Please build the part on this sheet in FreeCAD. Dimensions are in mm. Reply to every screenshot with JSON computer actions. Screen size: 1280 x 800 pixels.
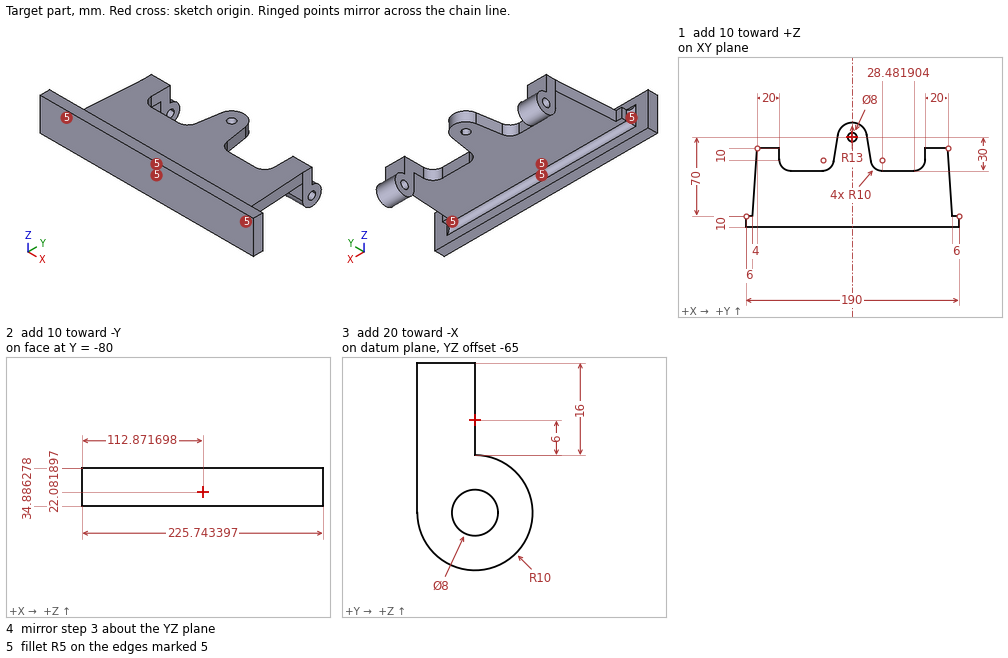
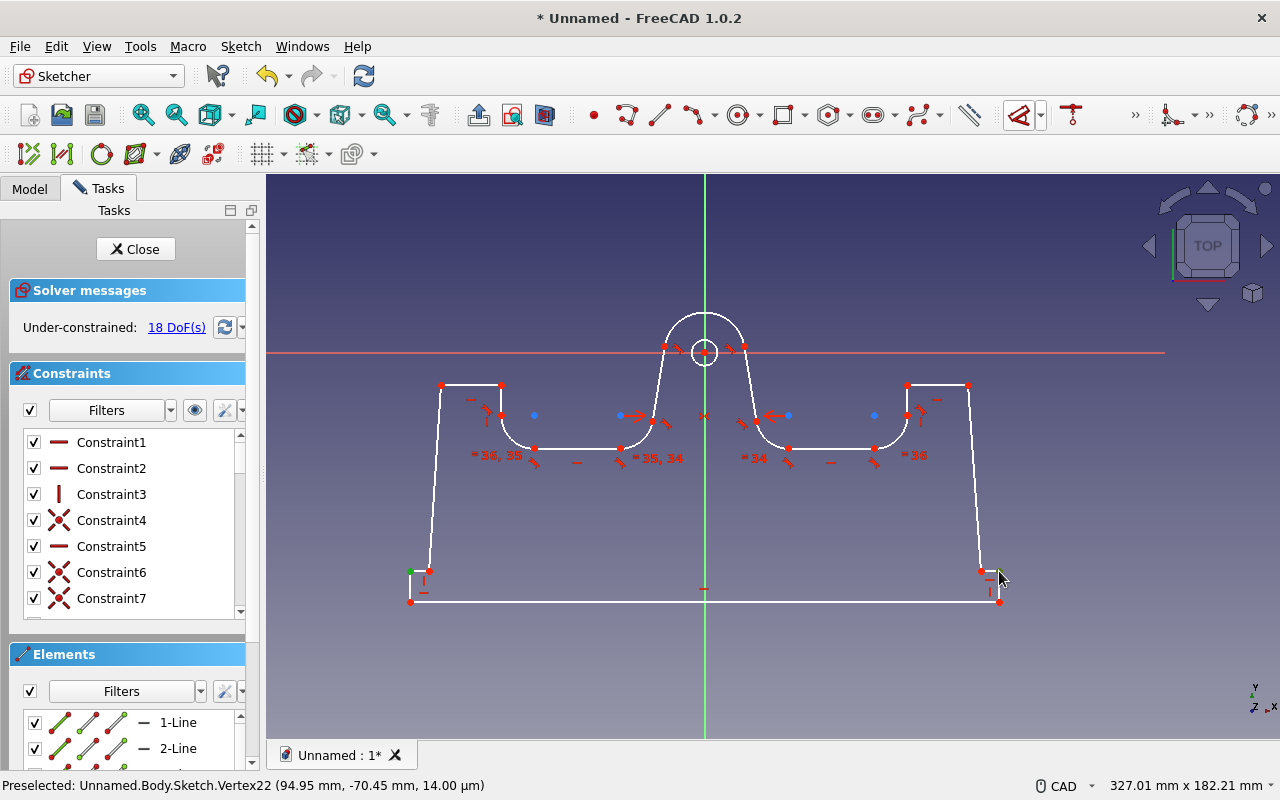
{"action": "left_click", "coordinate": [705, 675]}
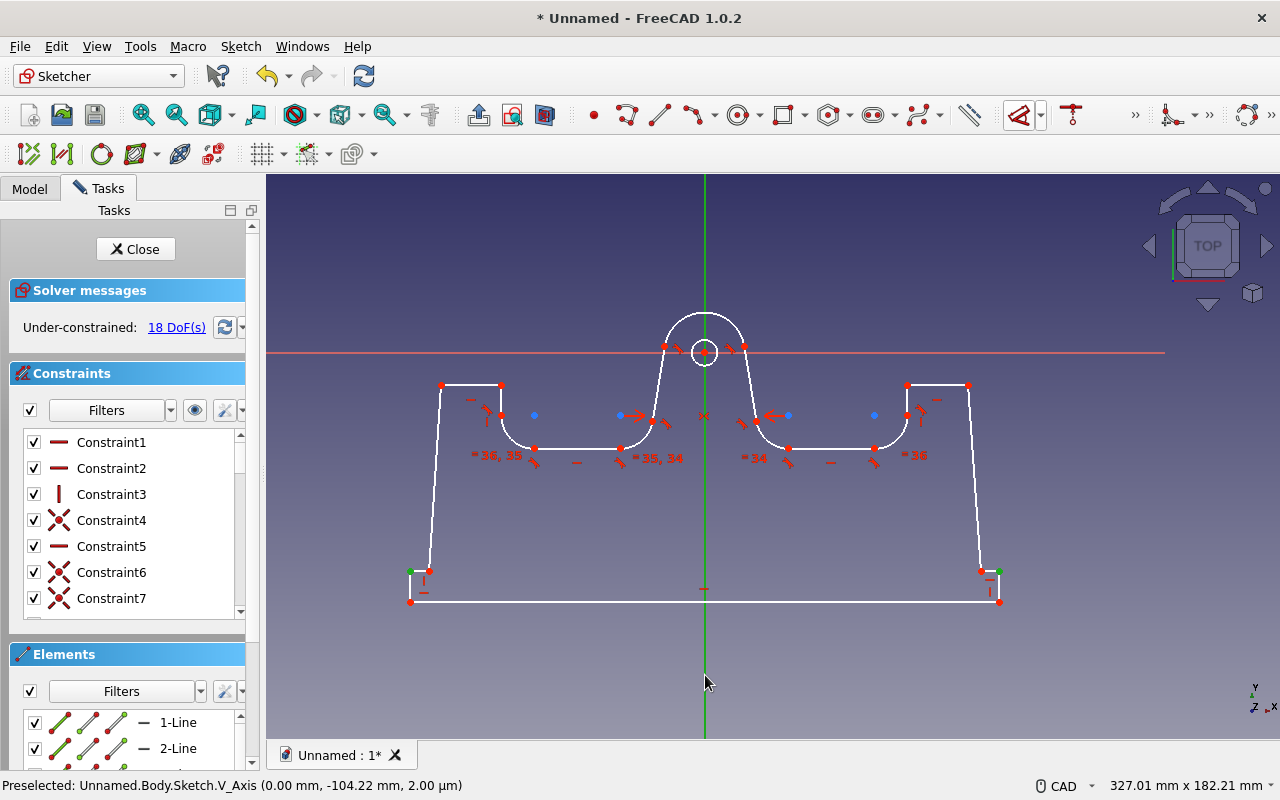
{"action": "key", "text": "s"}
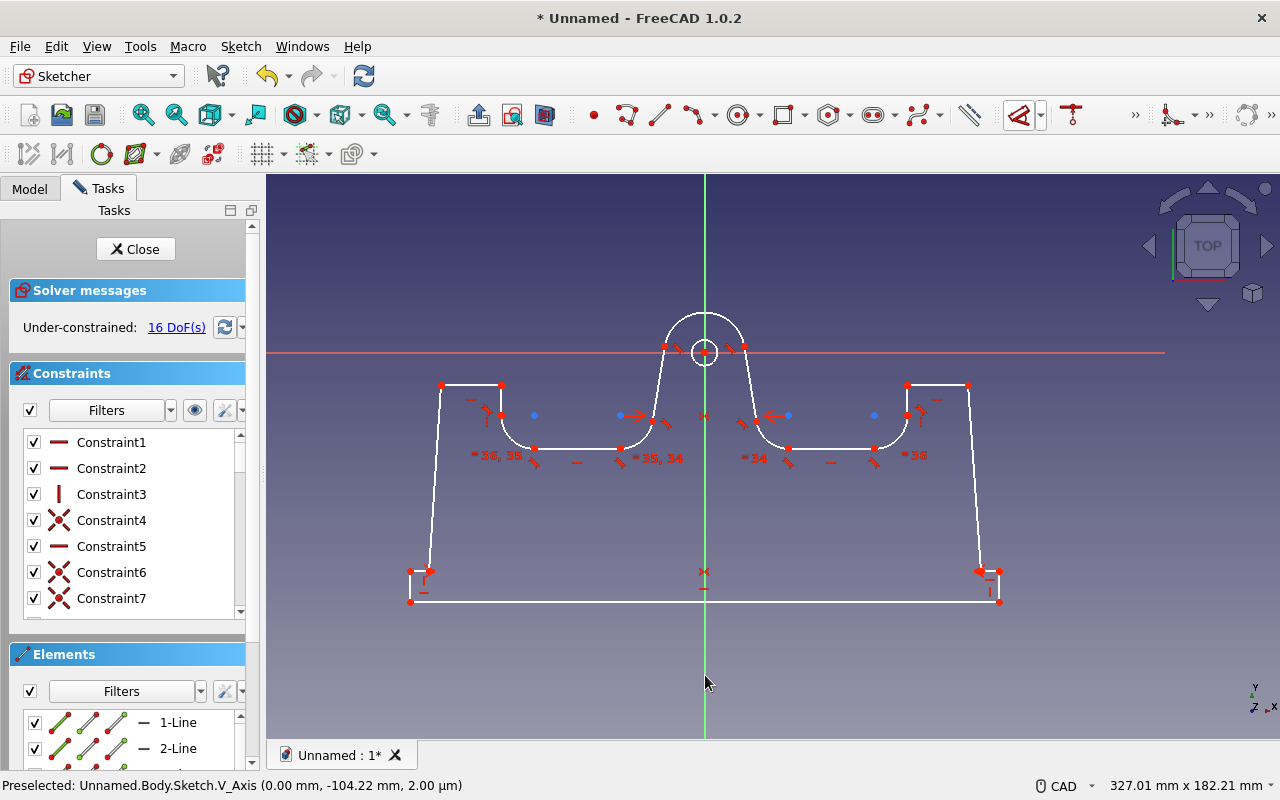
{"action": "left_click", "coordinate": [441, 385]}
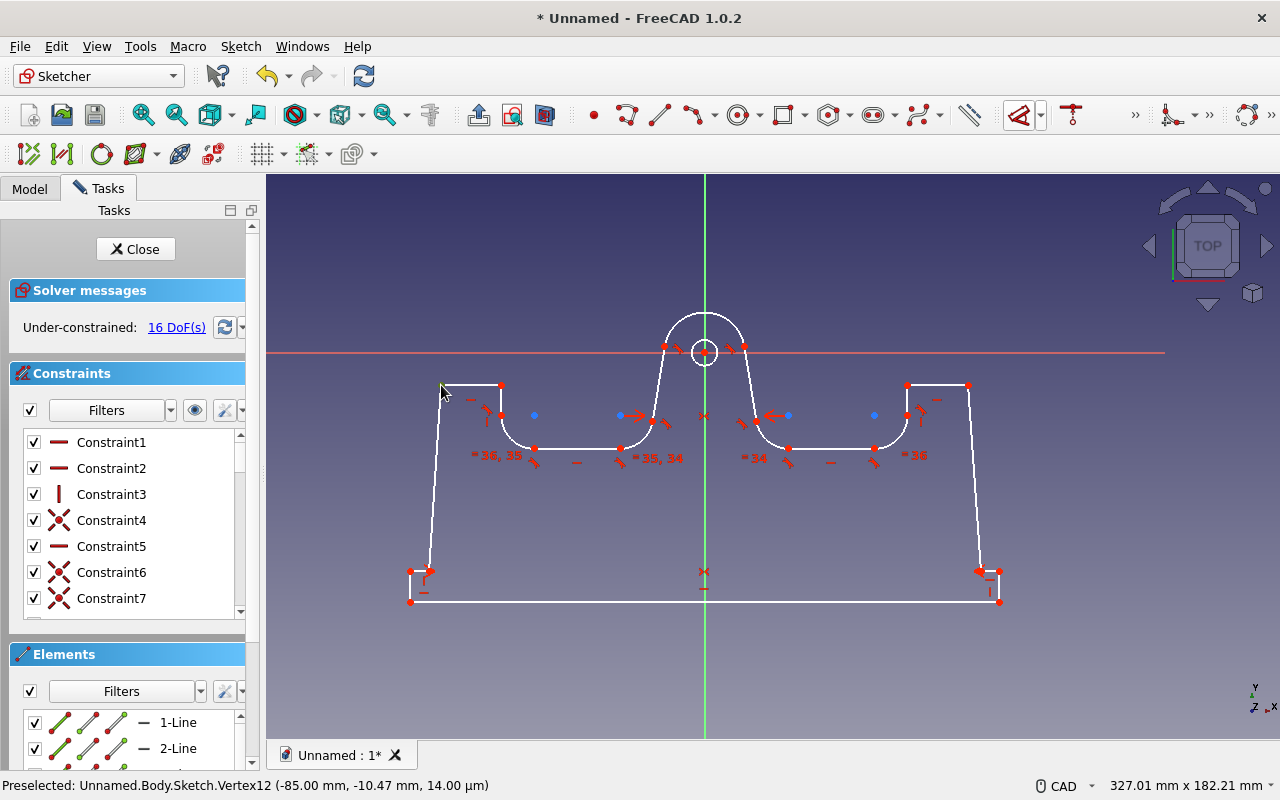
{"action": "left_click", "coordinate": [968, 385]}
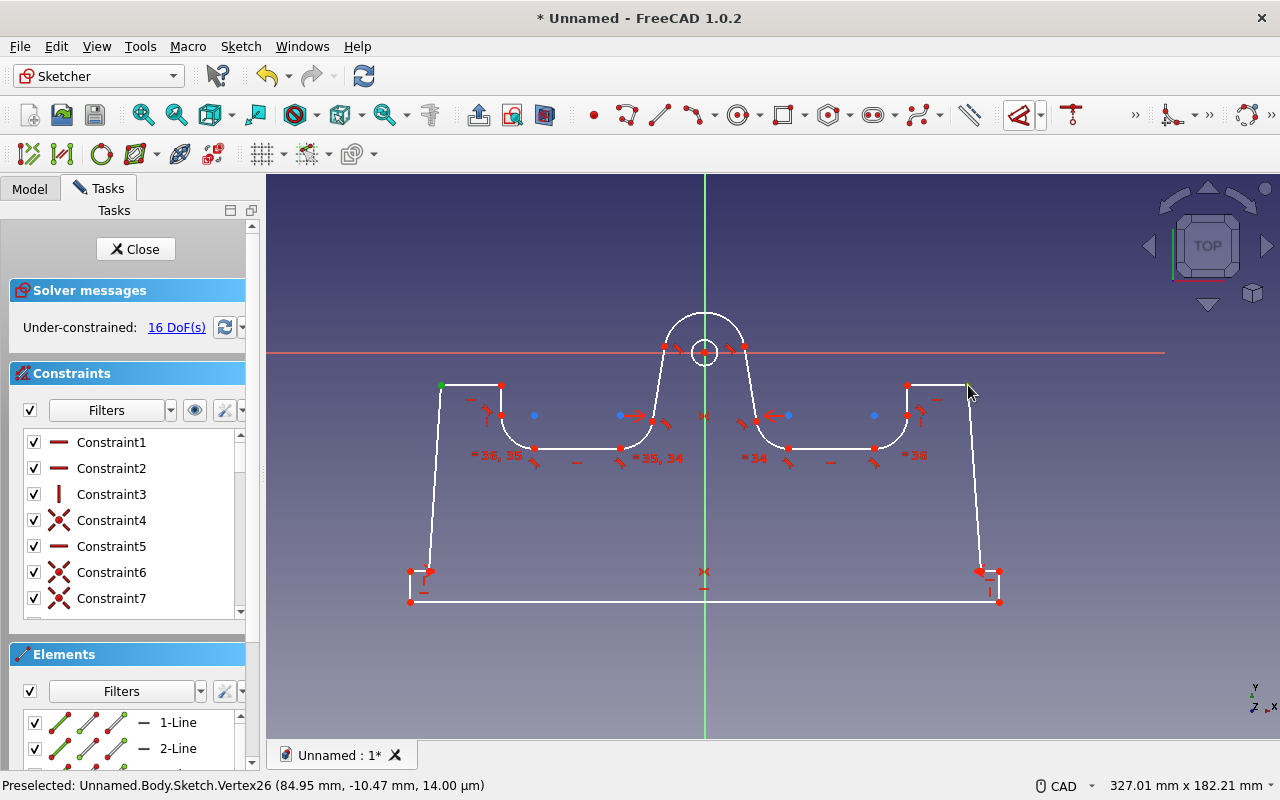
{"action": "left_click", "coordinate": [705, 675]}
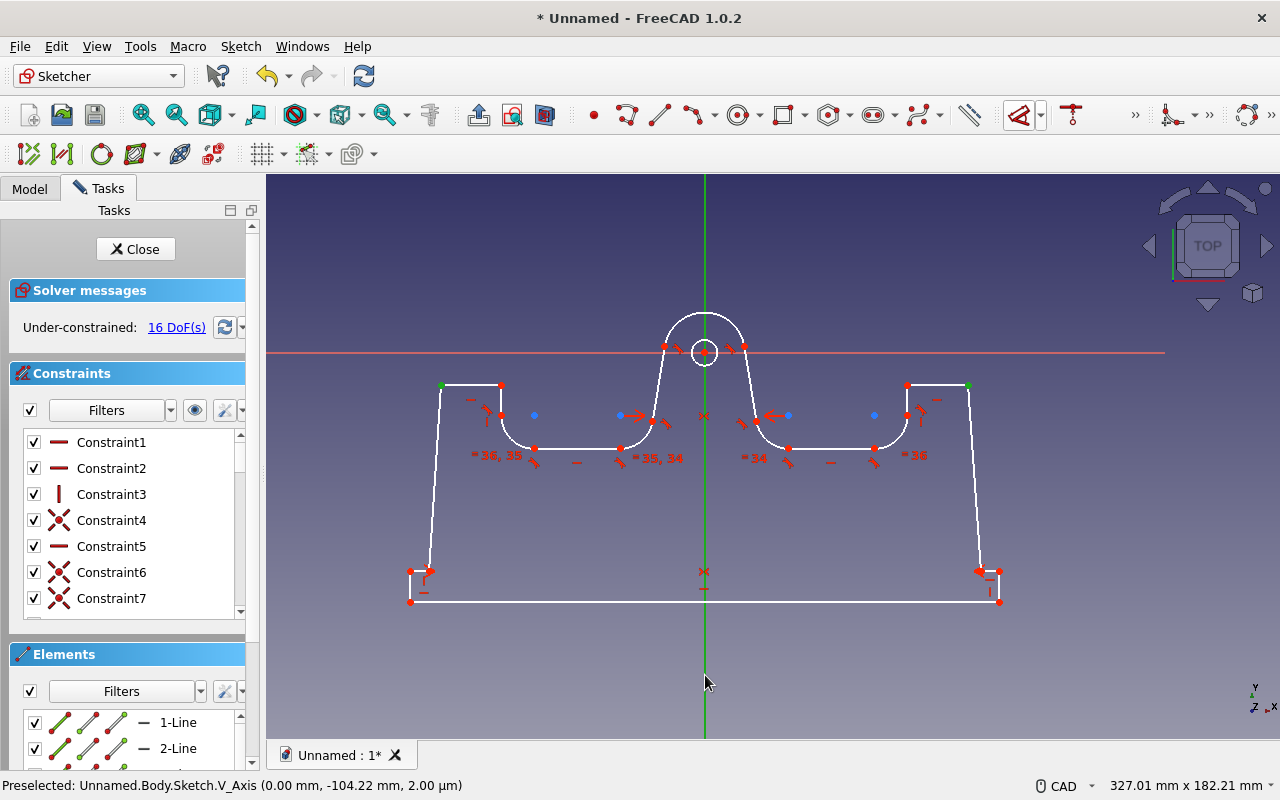
{"action": "key", "text": "s"}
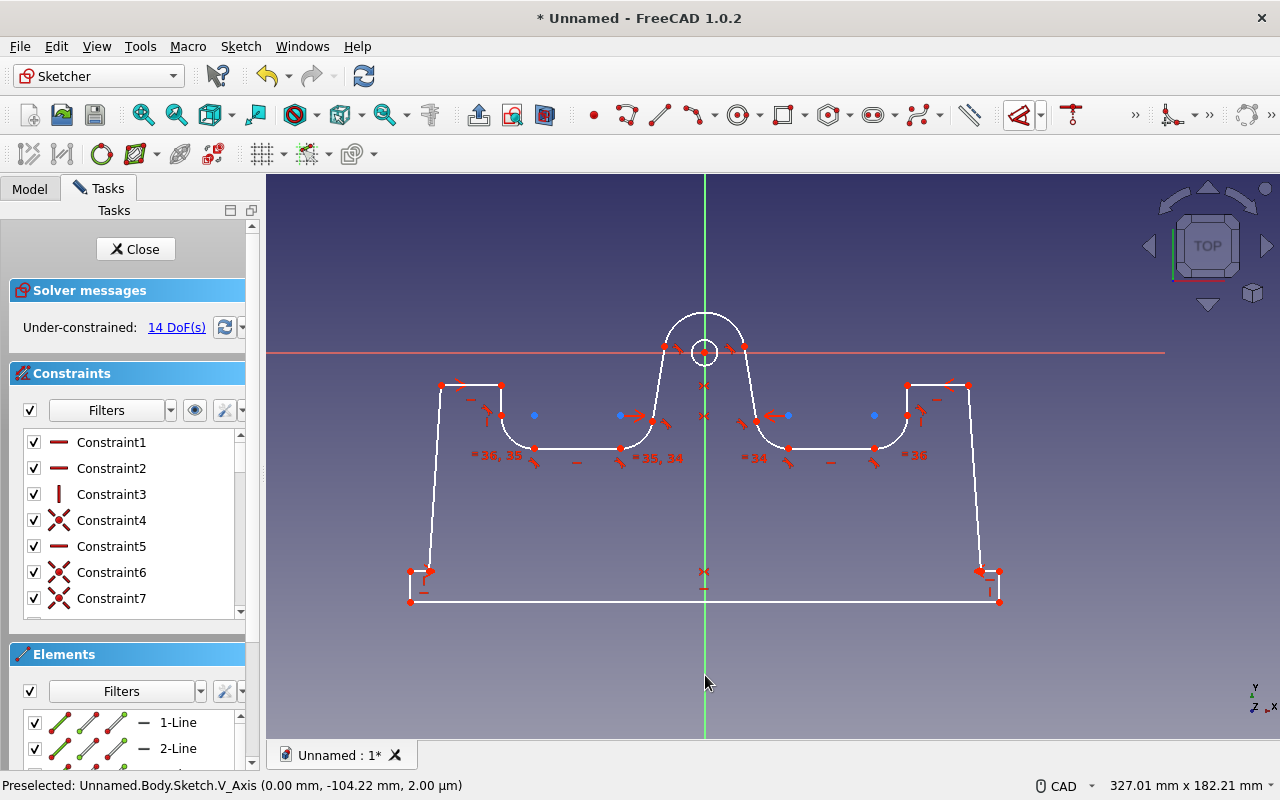
{"action": "left_click", "coordinate": [1018, 116]}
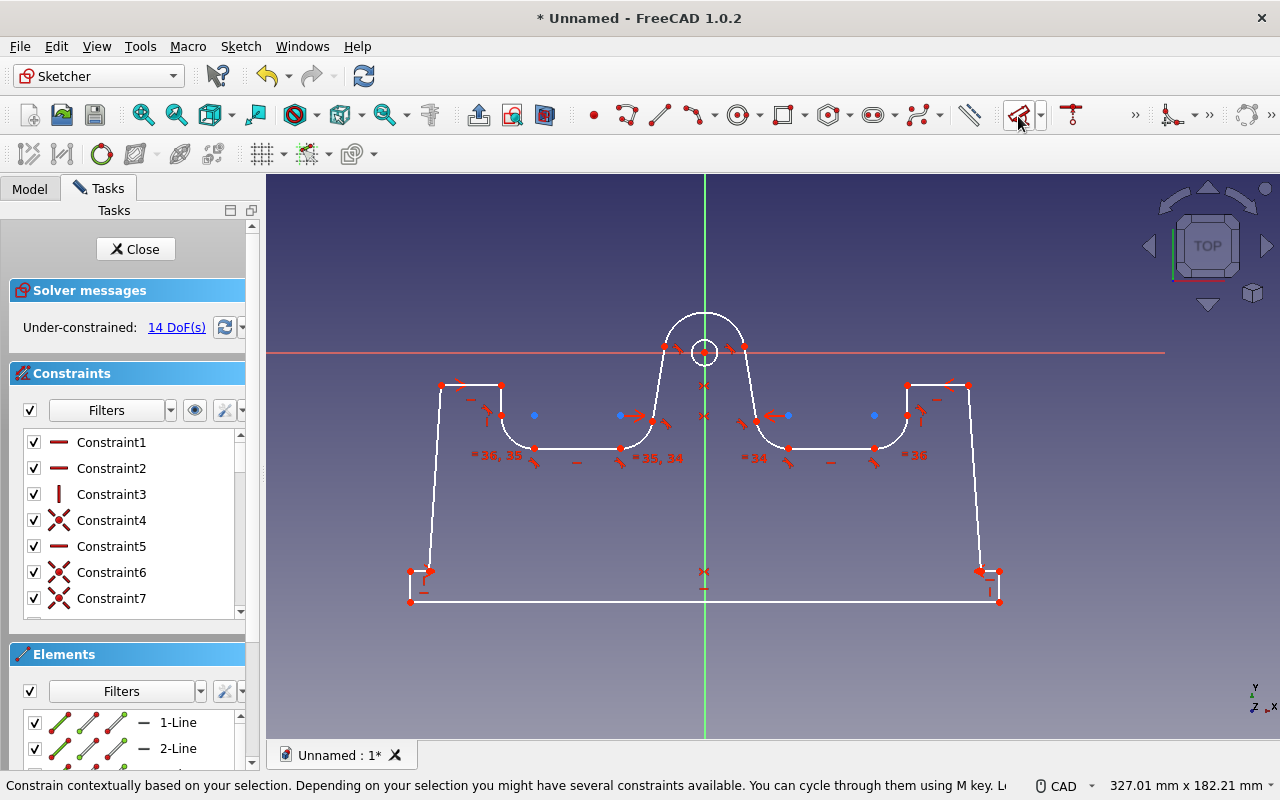
{"action": "scroll", "coordinate": [762, 434], "scroll_direction": "up", "scroll_amount": 2}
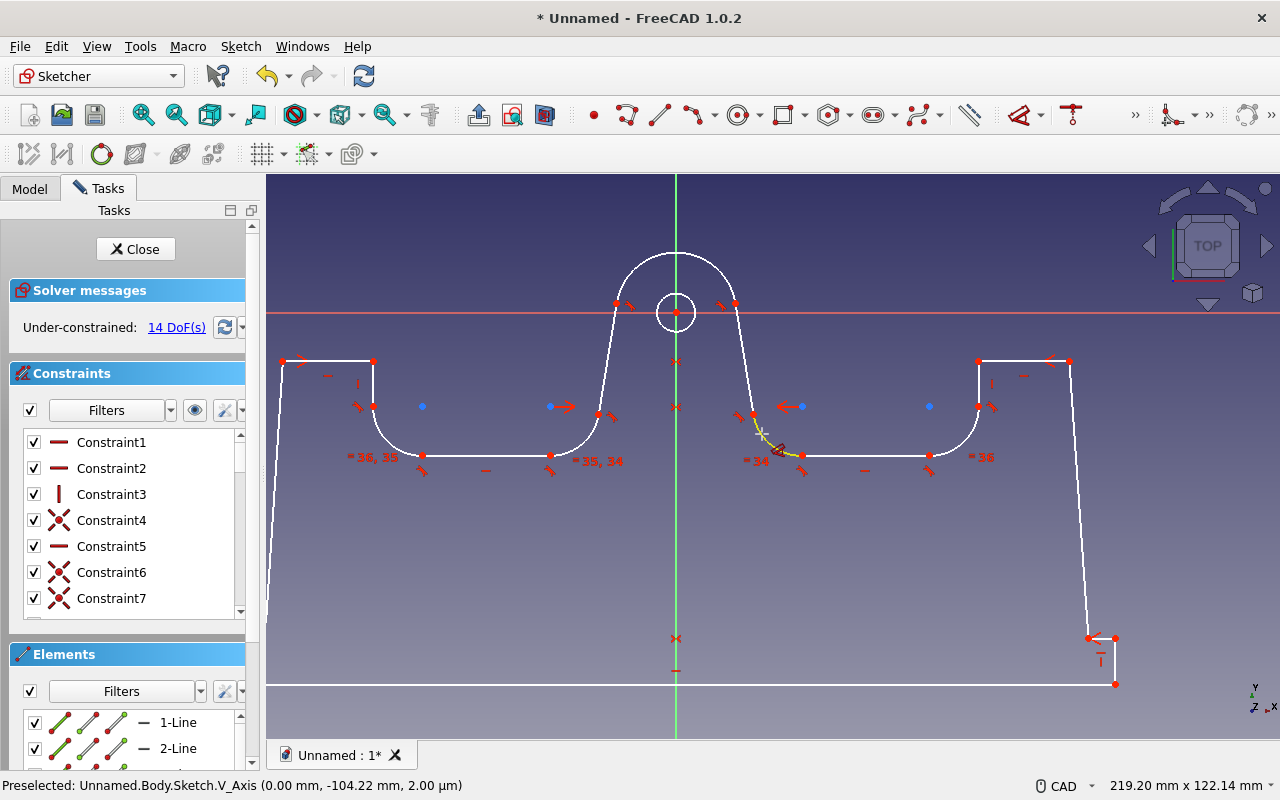
{"action": "left_click", "coordinate": [761, 434]}
{"action": "left_click", "coordinate": [734, 452]}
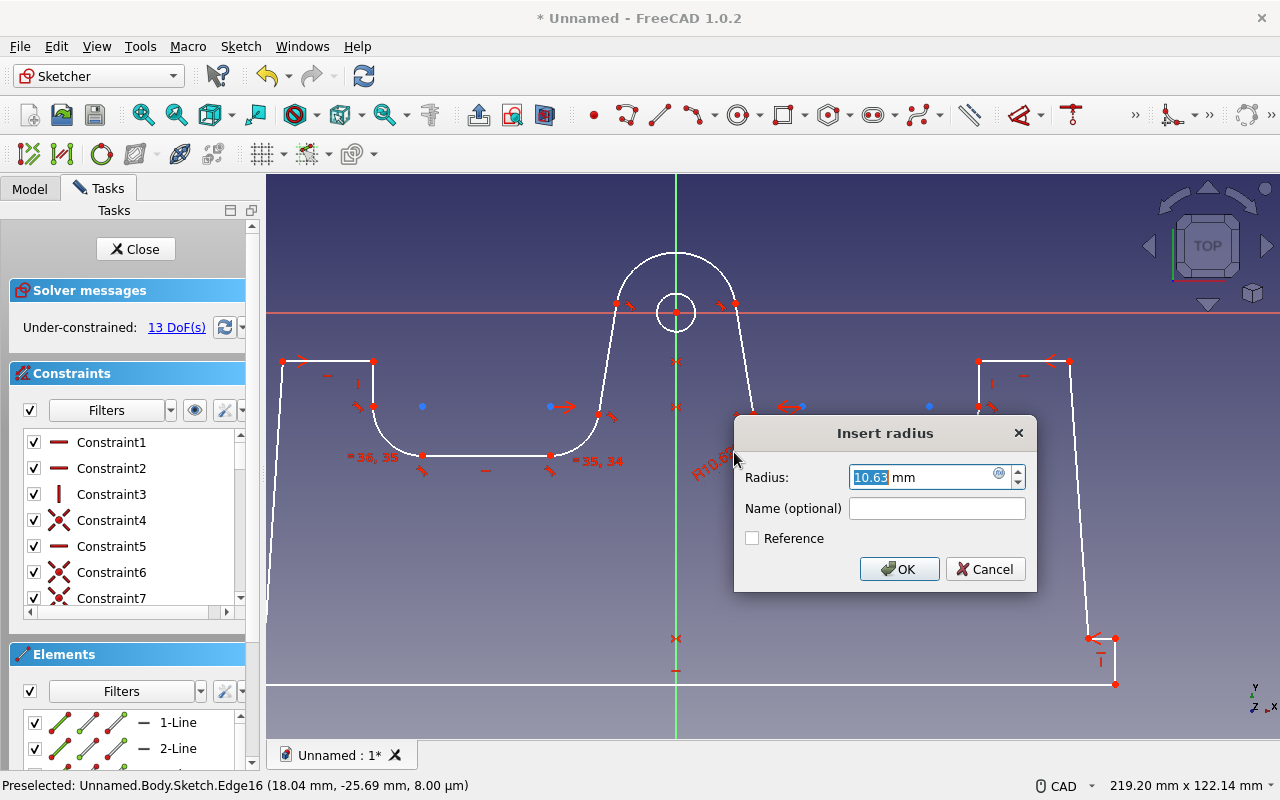
{"action": "type", "text": "10"}
{"action": "key", "text": "Return"}